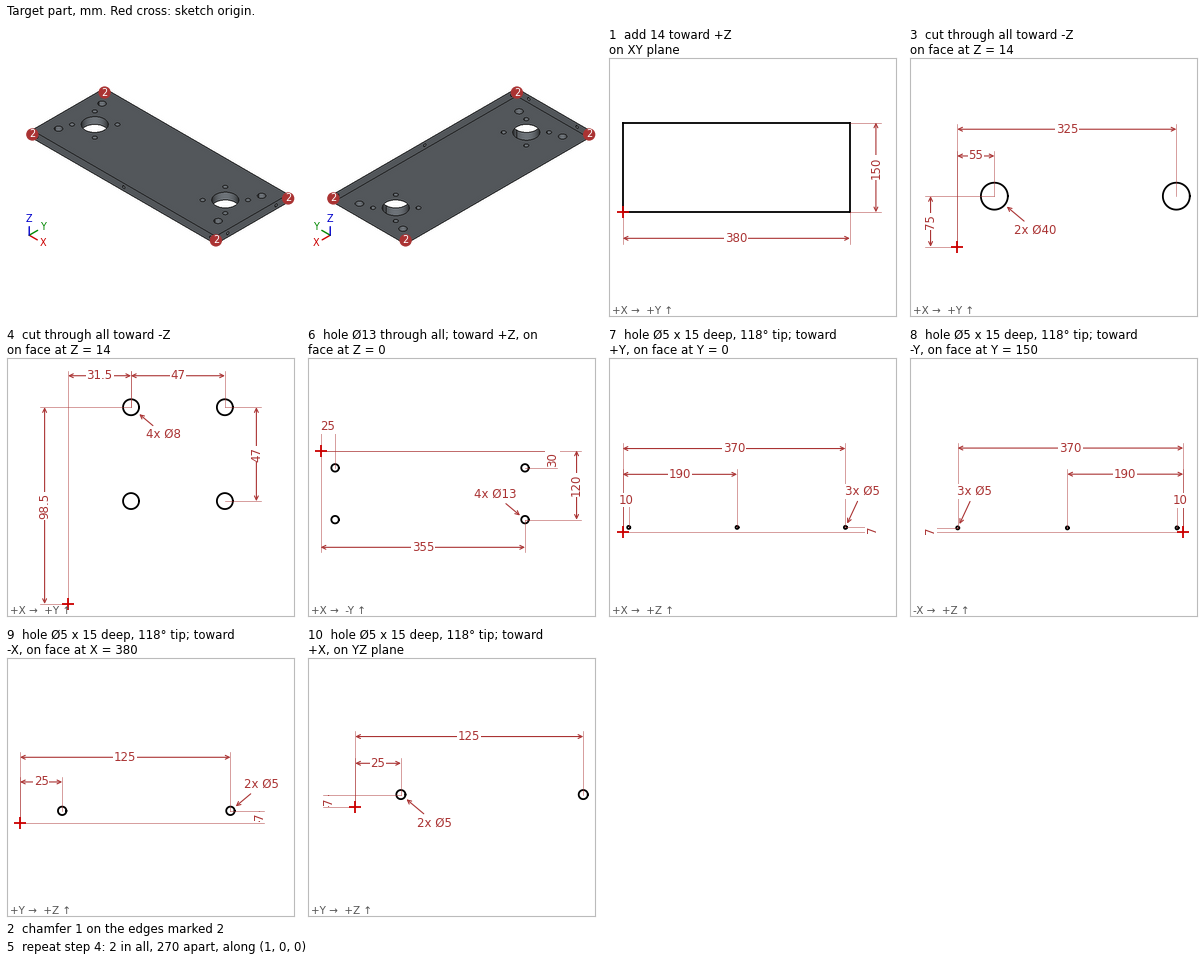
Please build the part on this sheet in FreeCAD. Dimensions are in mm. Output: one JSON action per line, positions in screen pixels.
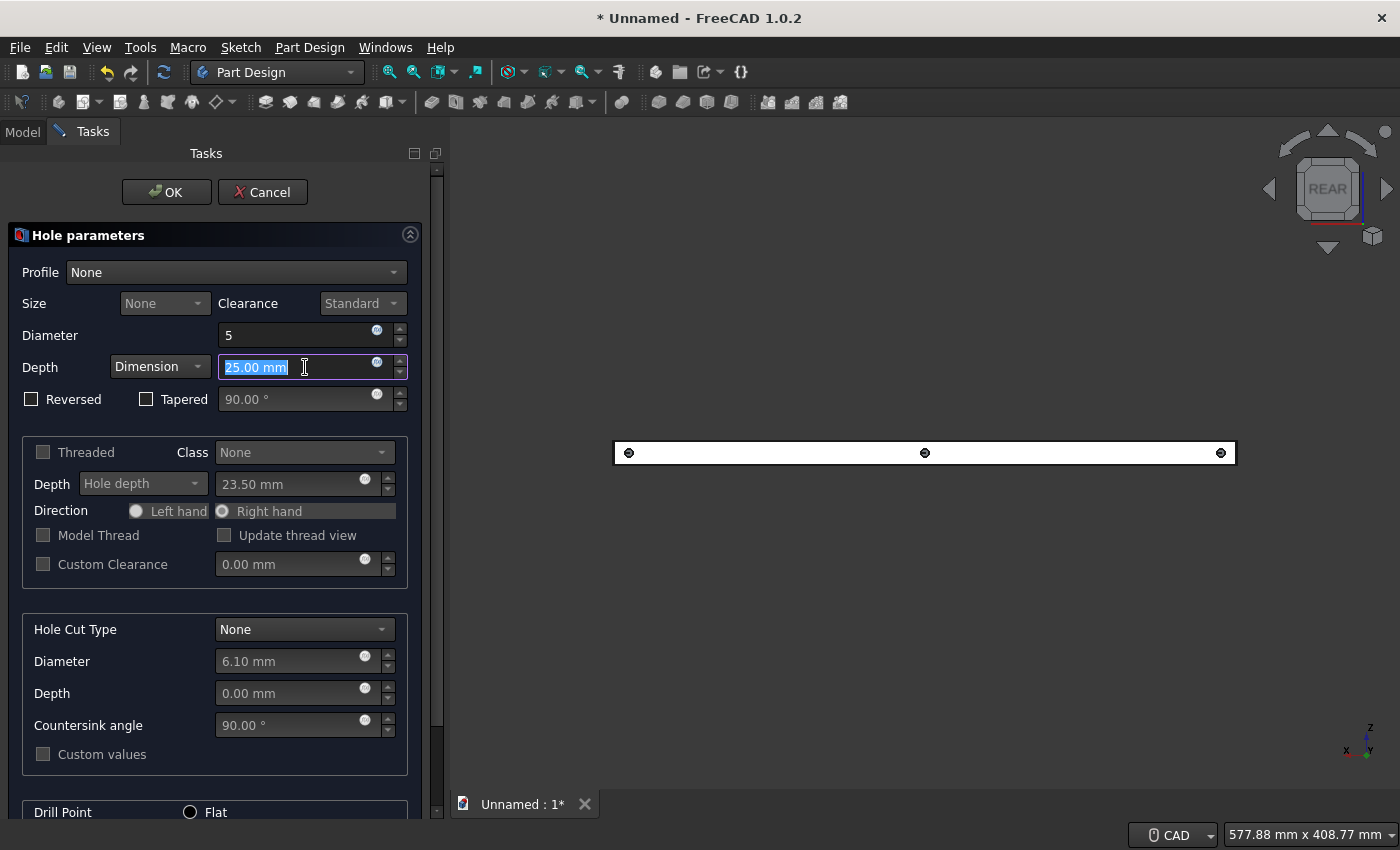
{"action": "type", "text": "15"}
{"action": "key", "text": "Tab"}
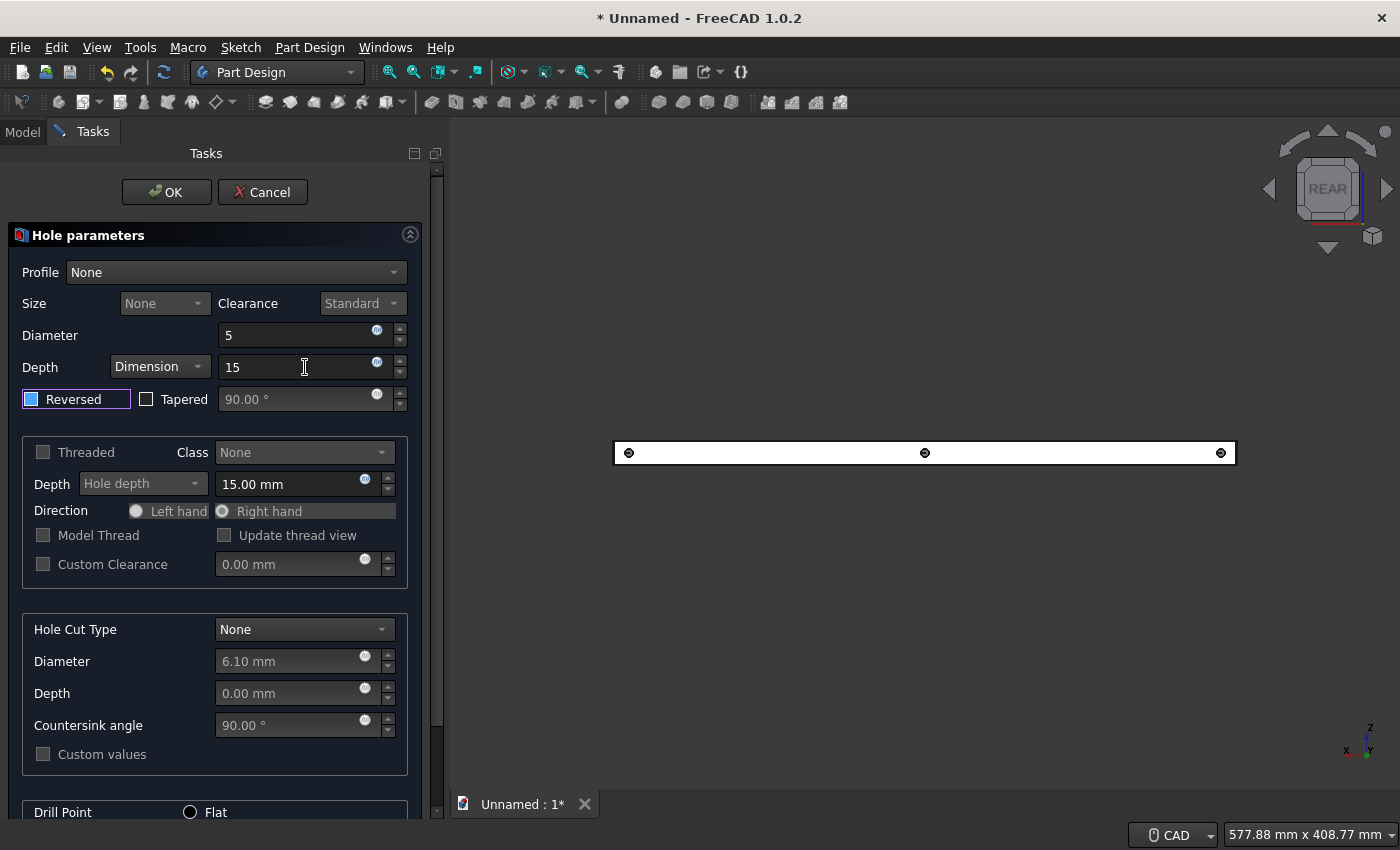
{"action": "left_click", "coordinate": [167, 192]}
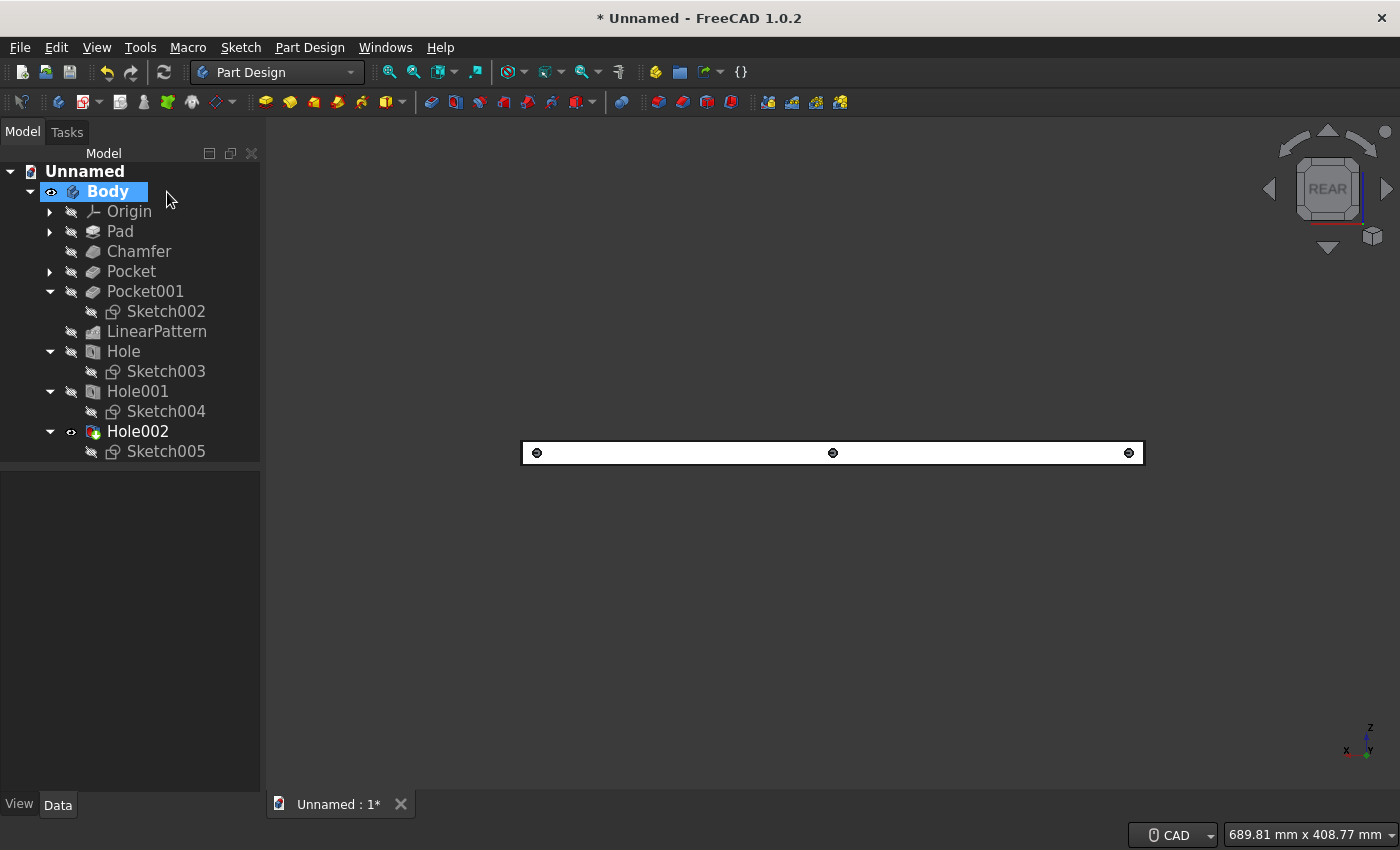
{"action": "key", "text": "0"}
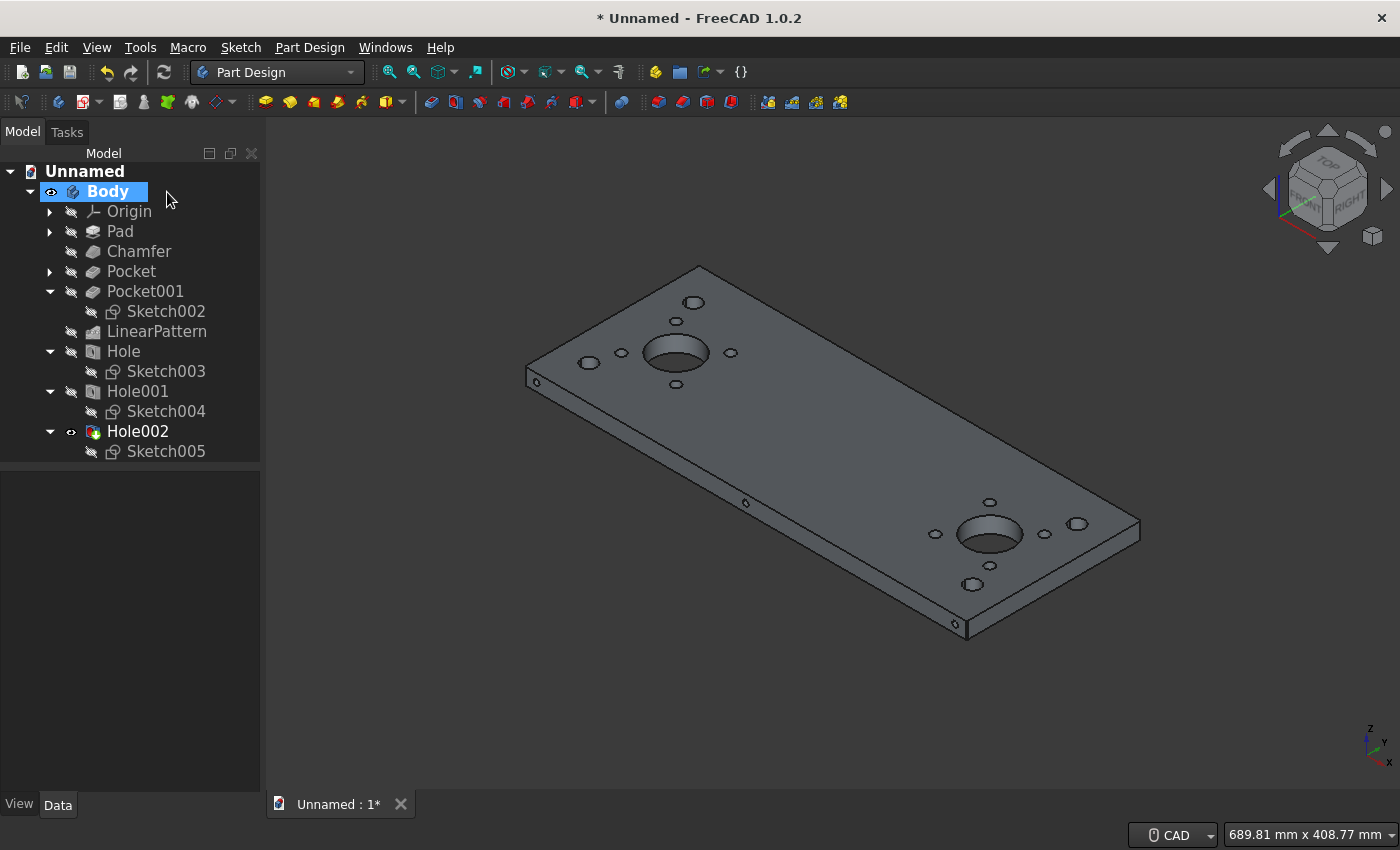
{"action": "key", "text": "3"}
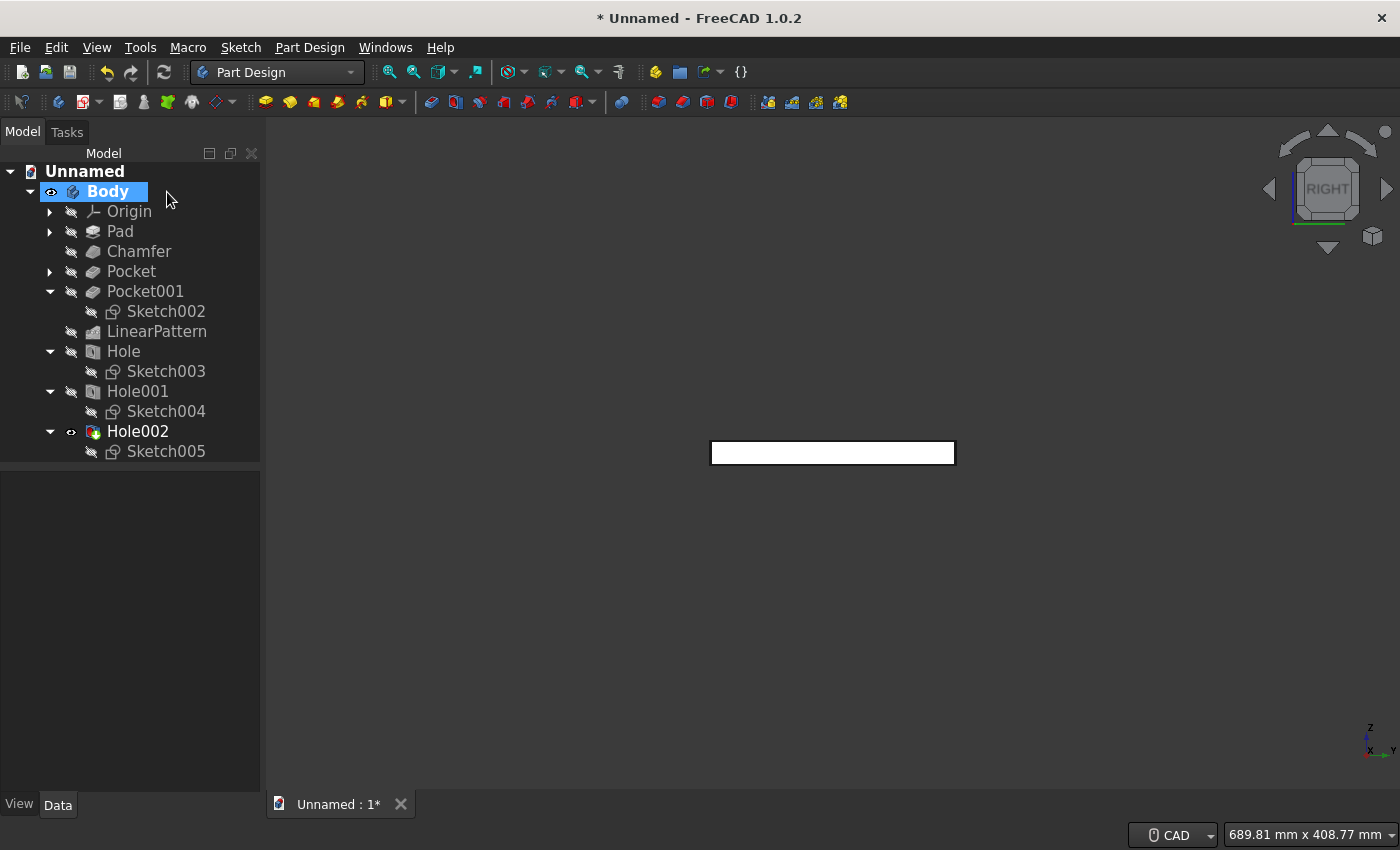
{"action": "left_click", "coordinate": [390, 72]}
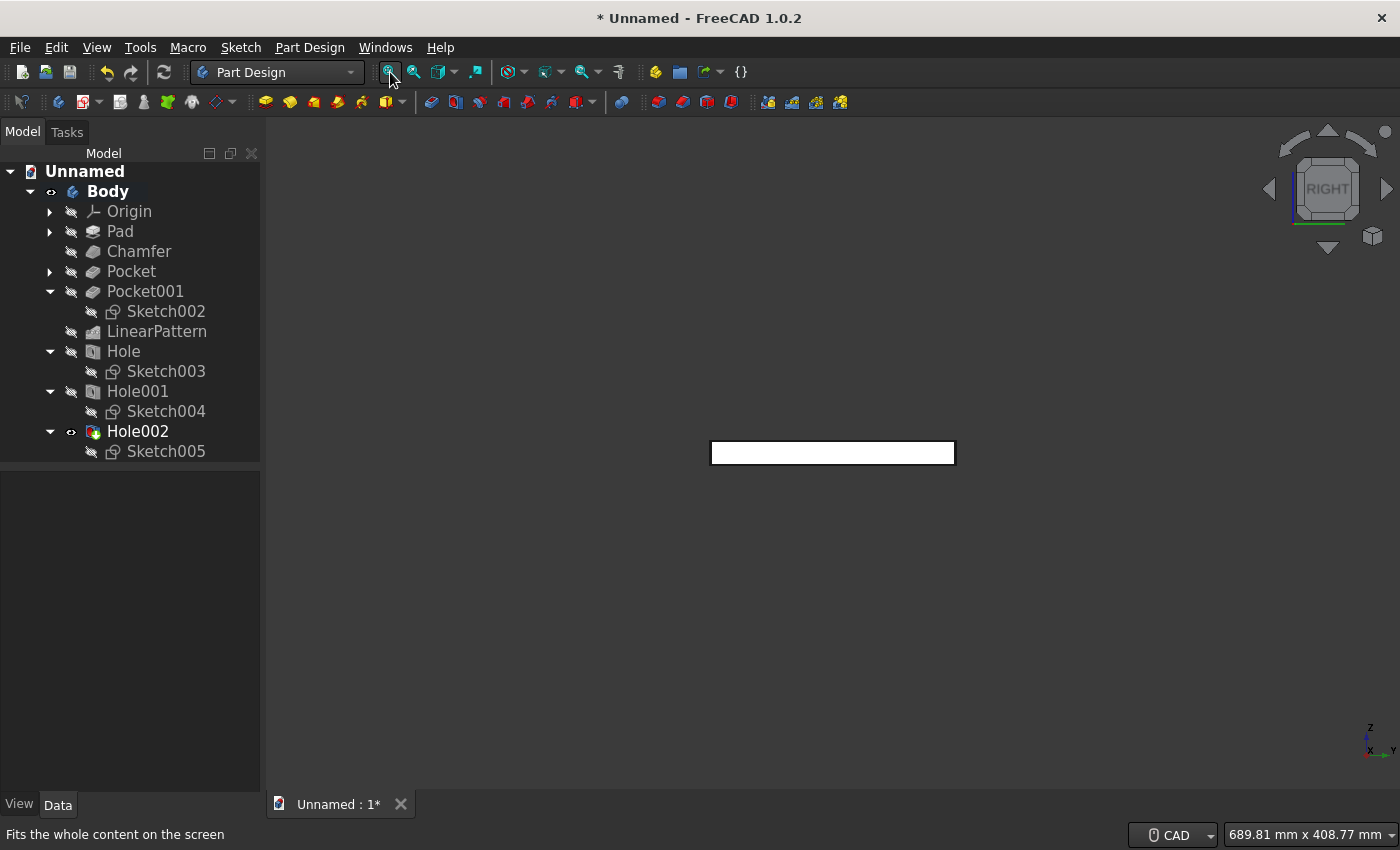
{"action": "left_click", "coordinate": [937, 452]}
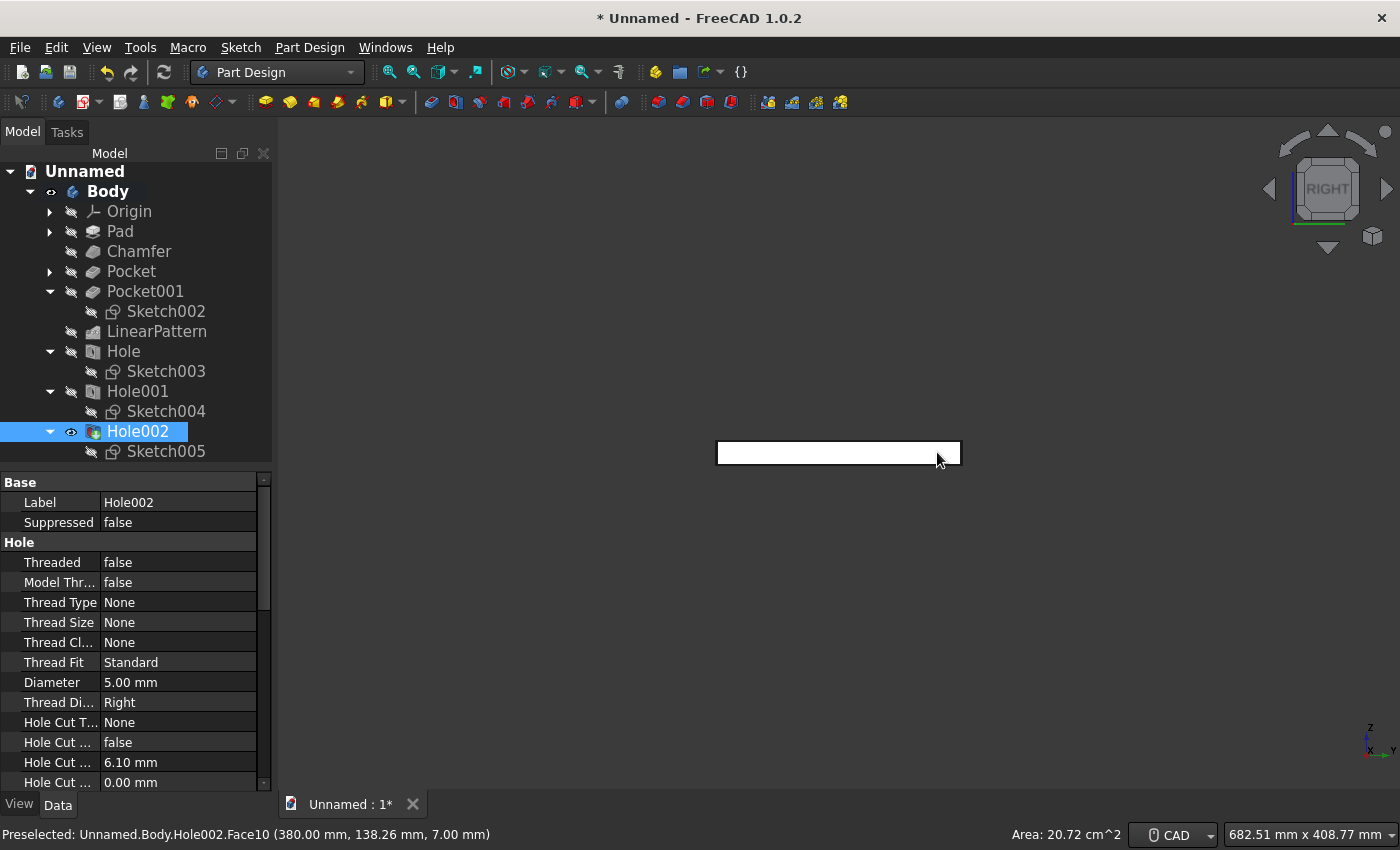
{"action": "left_click", "coordinate": [84, 102]}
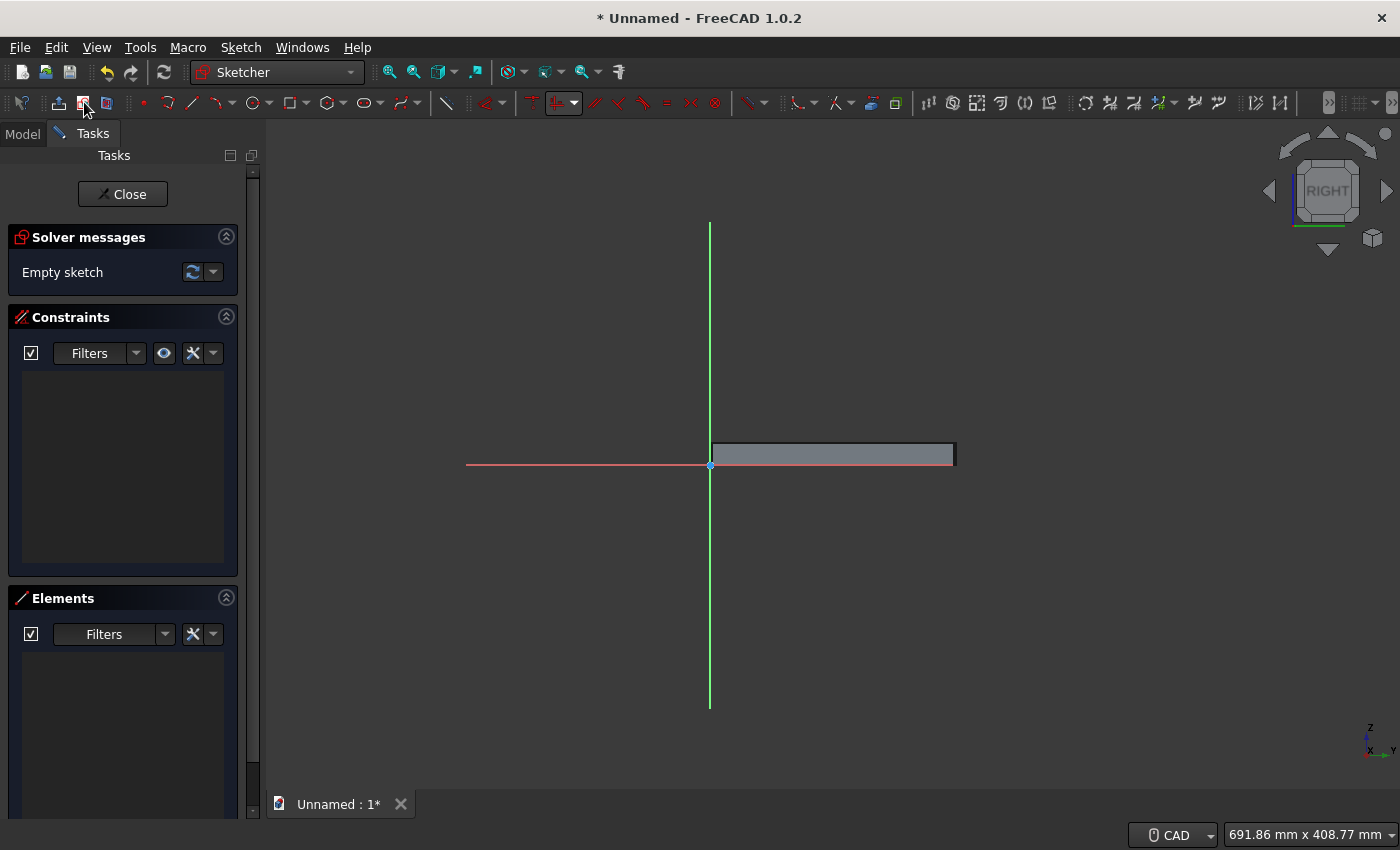
{"action": "scroll", "coordinate": [836, 459], "scroll_direction": "up", "scroll_amount": 6}